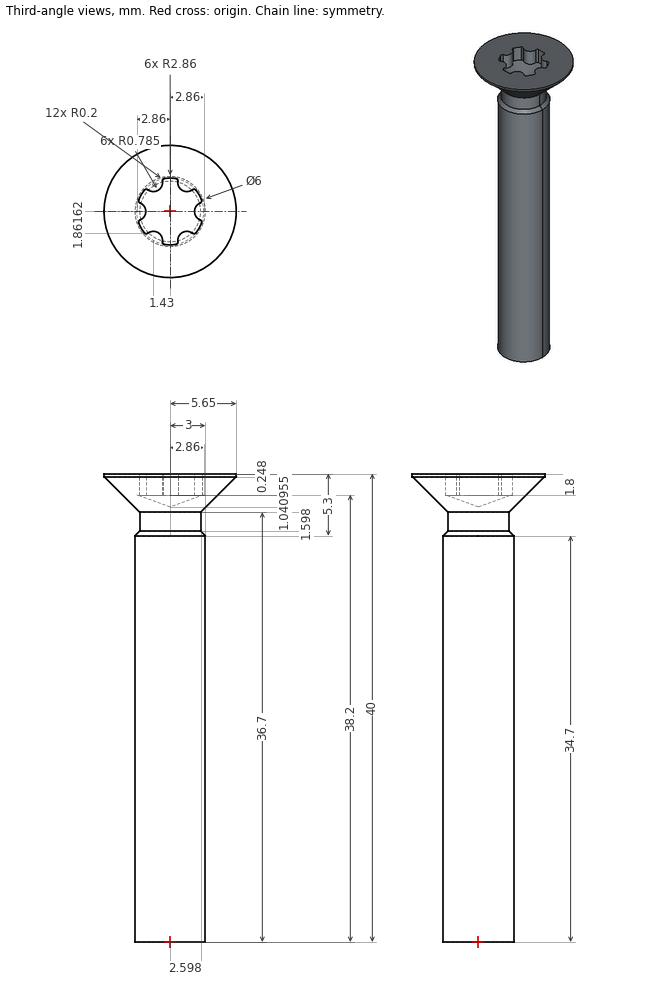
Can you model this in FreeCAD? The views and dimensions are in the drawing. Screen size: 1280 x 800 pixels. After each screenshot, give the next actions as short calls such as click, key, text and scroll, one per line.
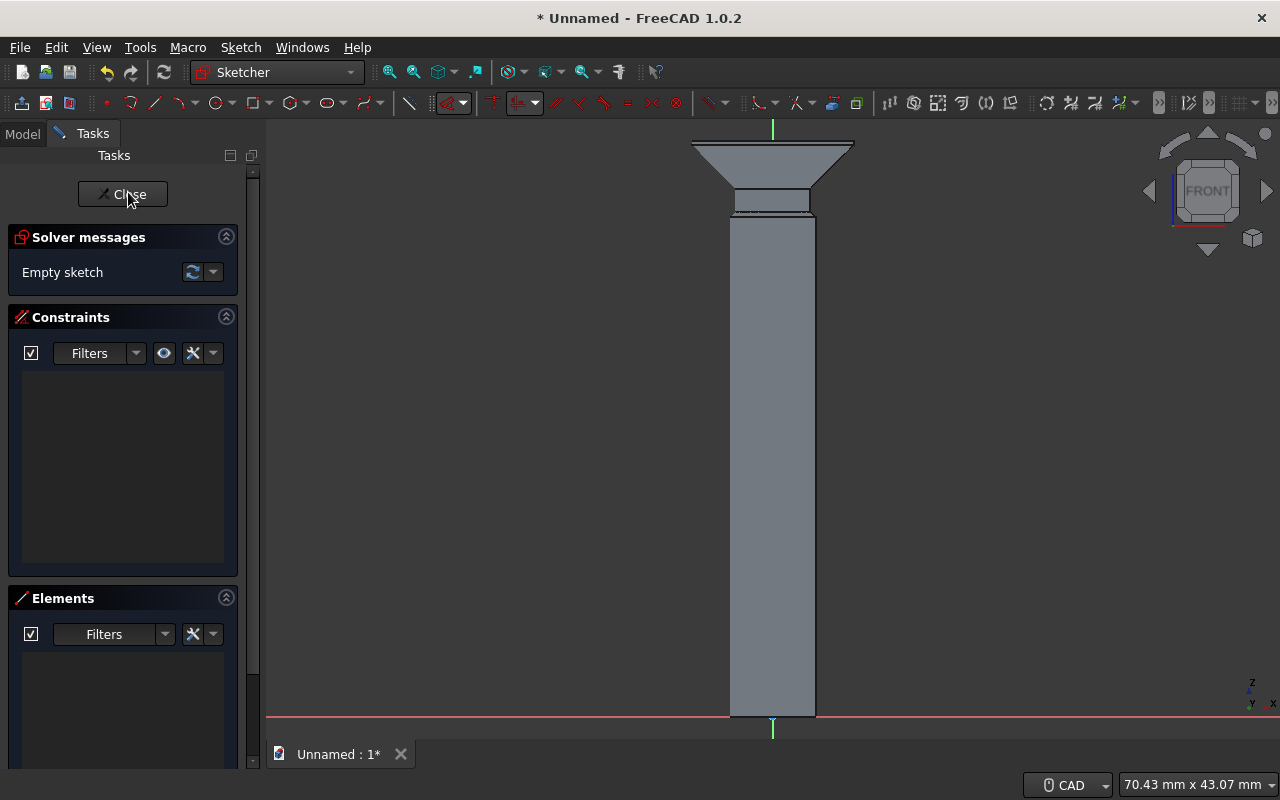
click(70, 104)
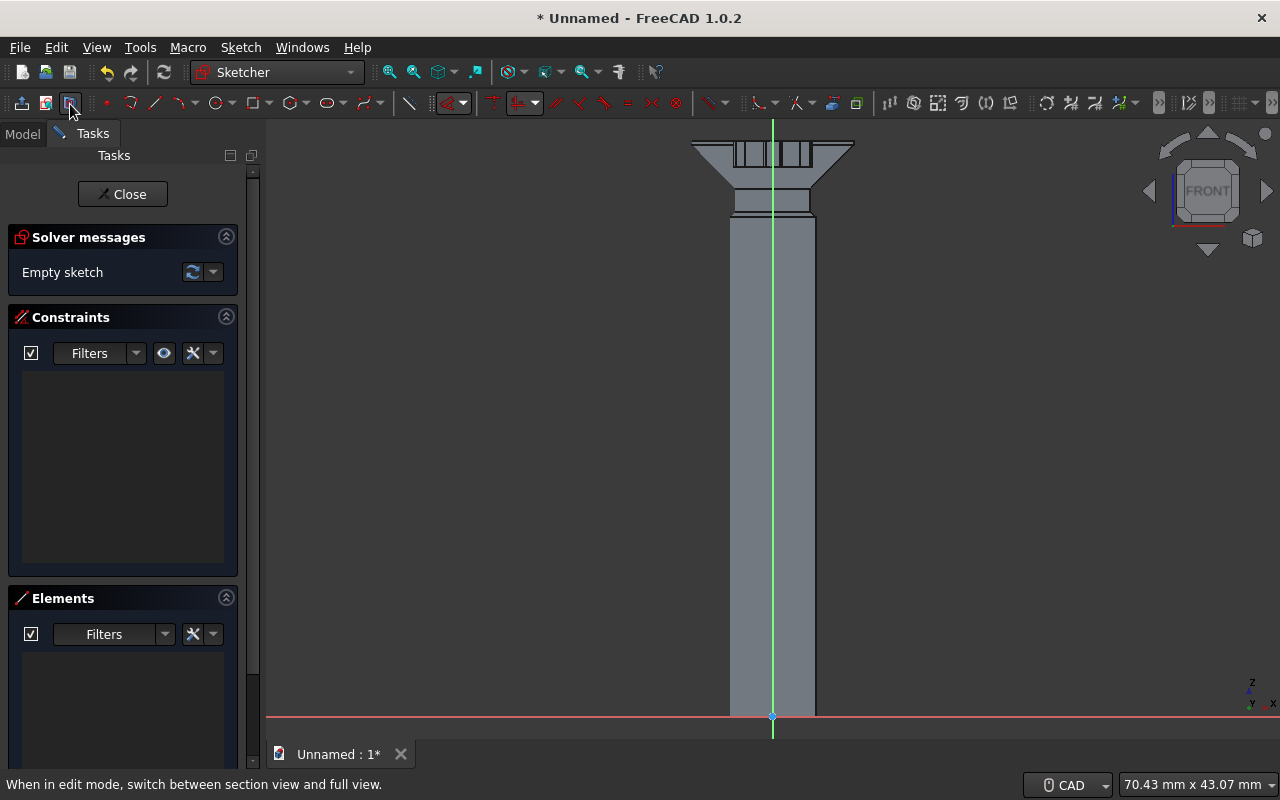
scroll(801, 154, up, 13)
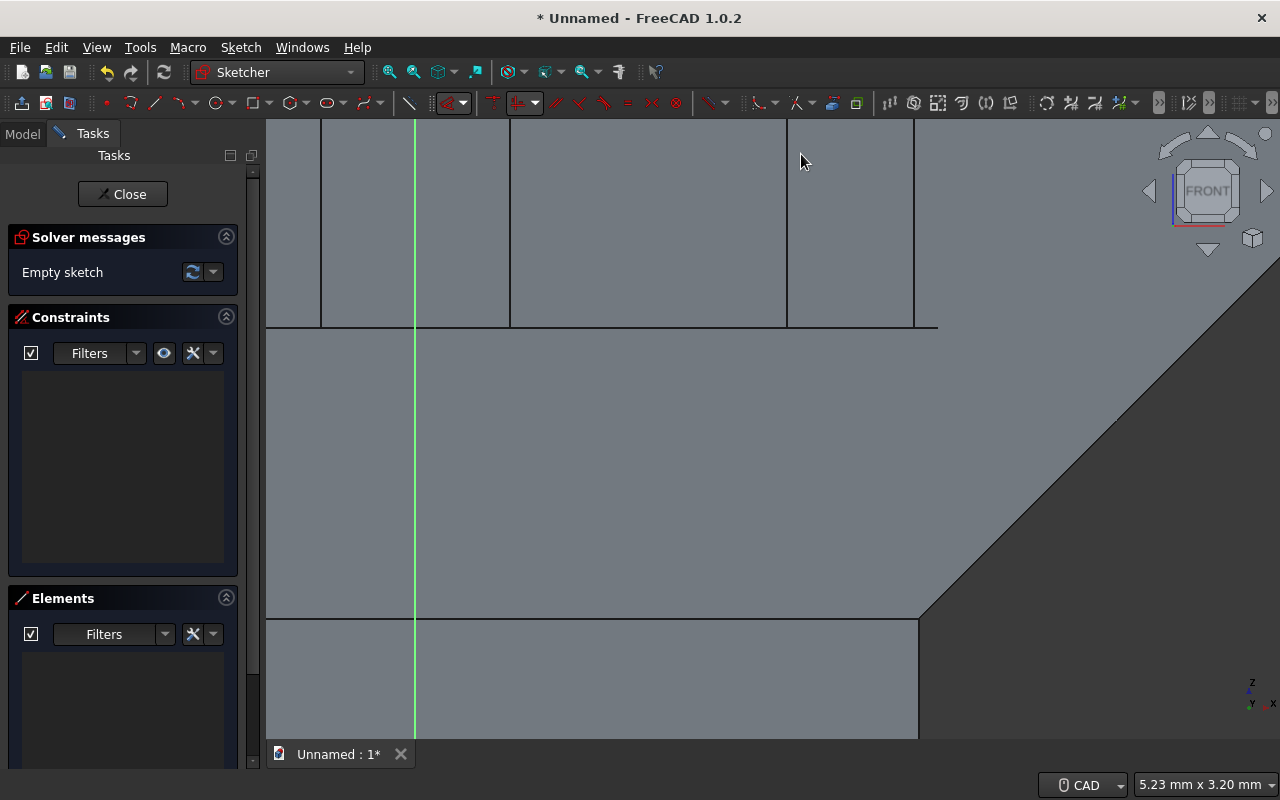
key(g)
key(m)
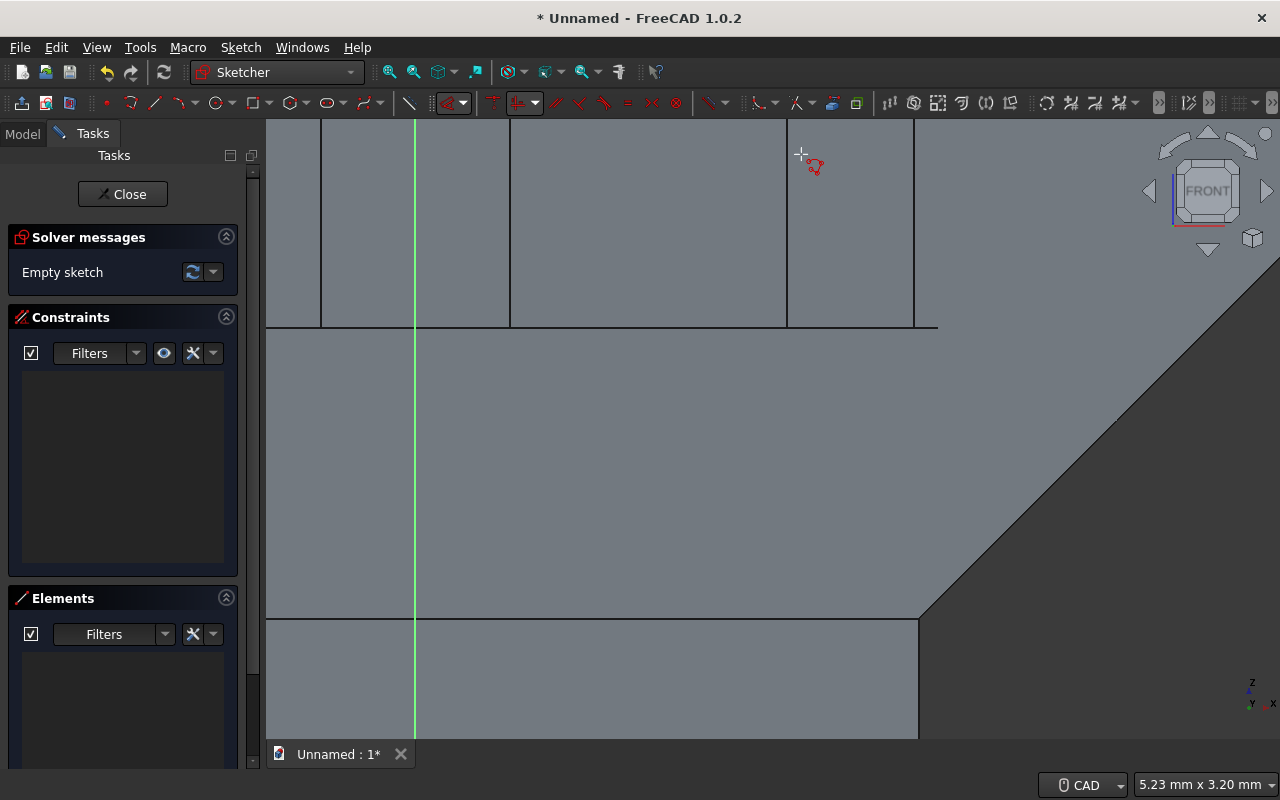
click(415, 530)
click(424, 328)
click(970, 328)
click(415, 531)
key(Escape)
key(Escape)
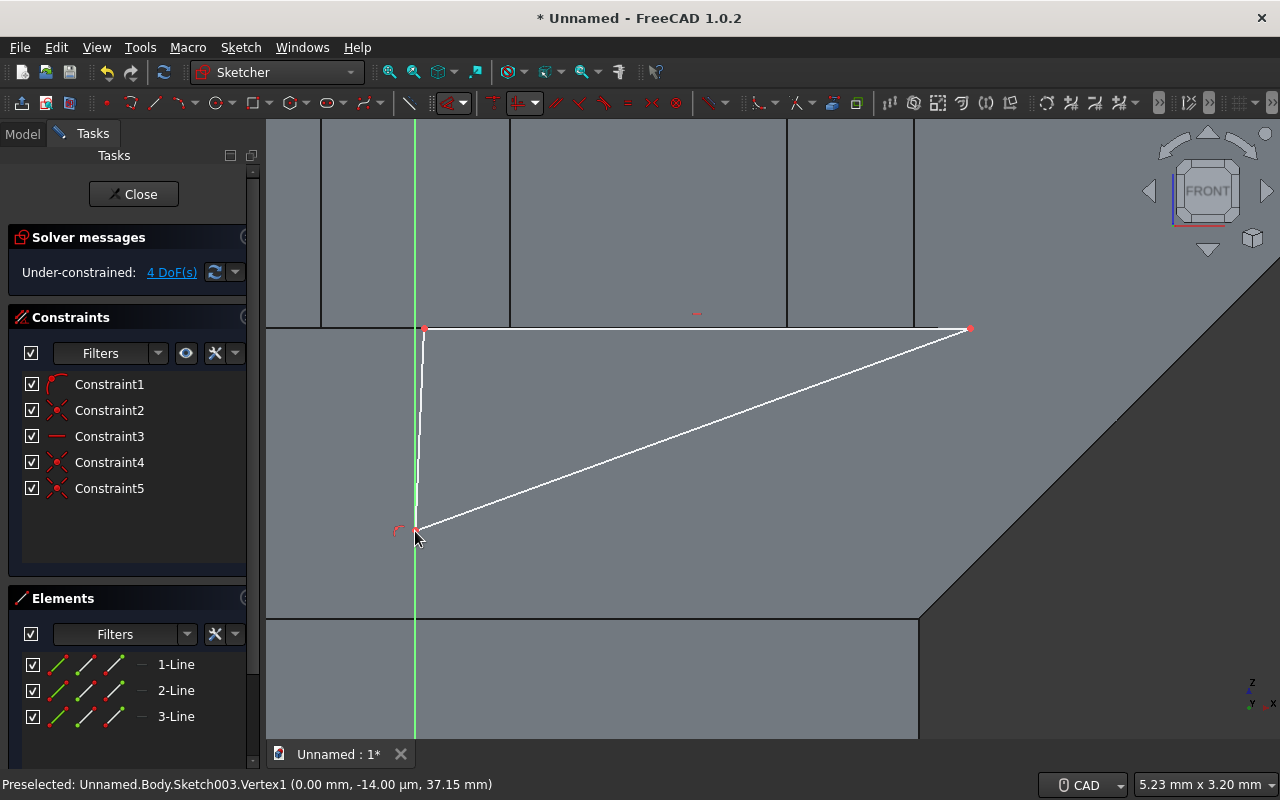
click(418, 470)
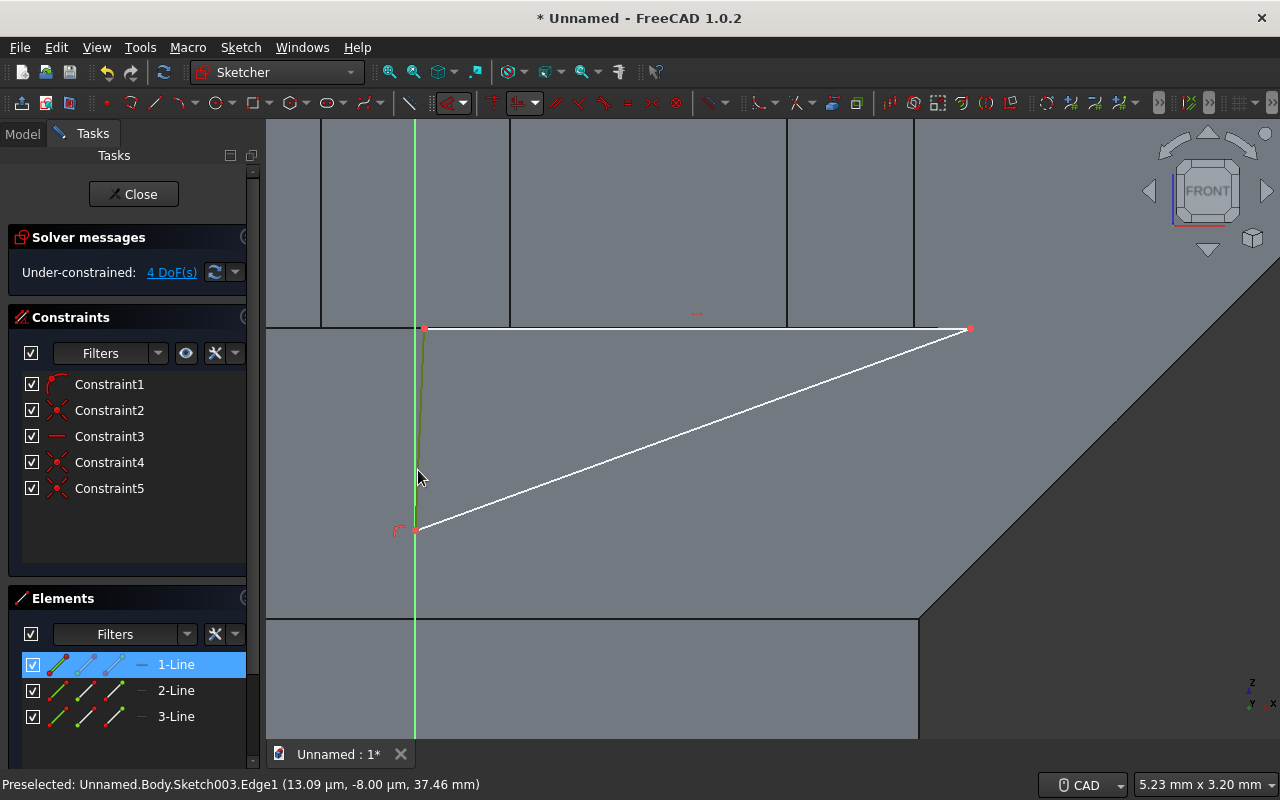
click(538, 104)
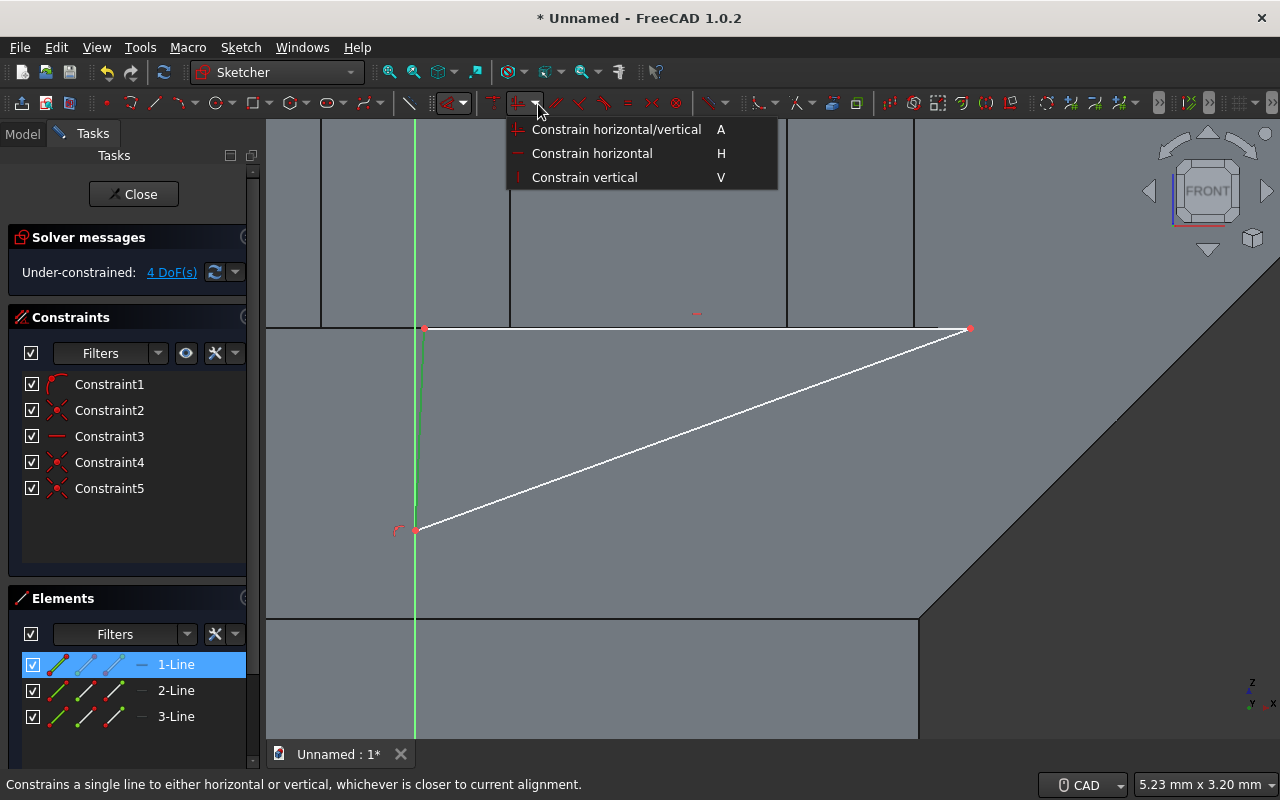
click(642, 177)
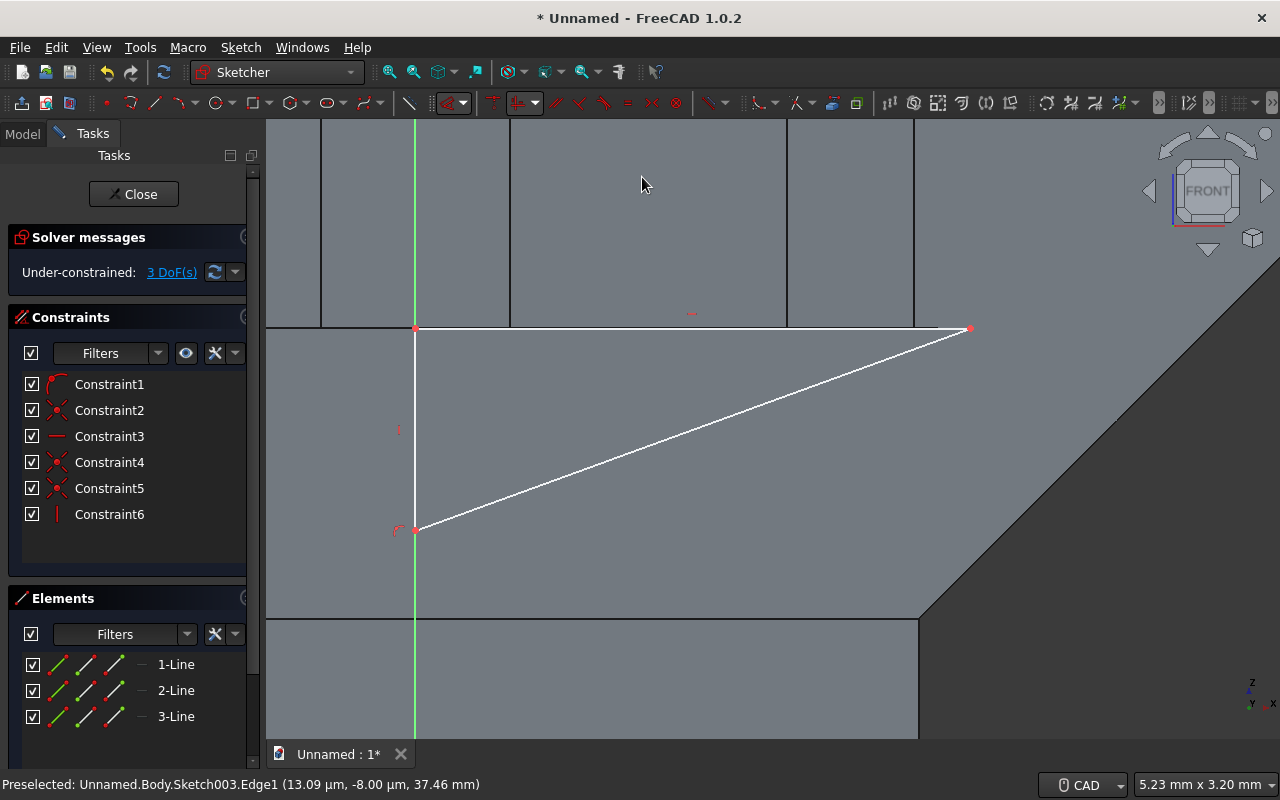
click(582, 329)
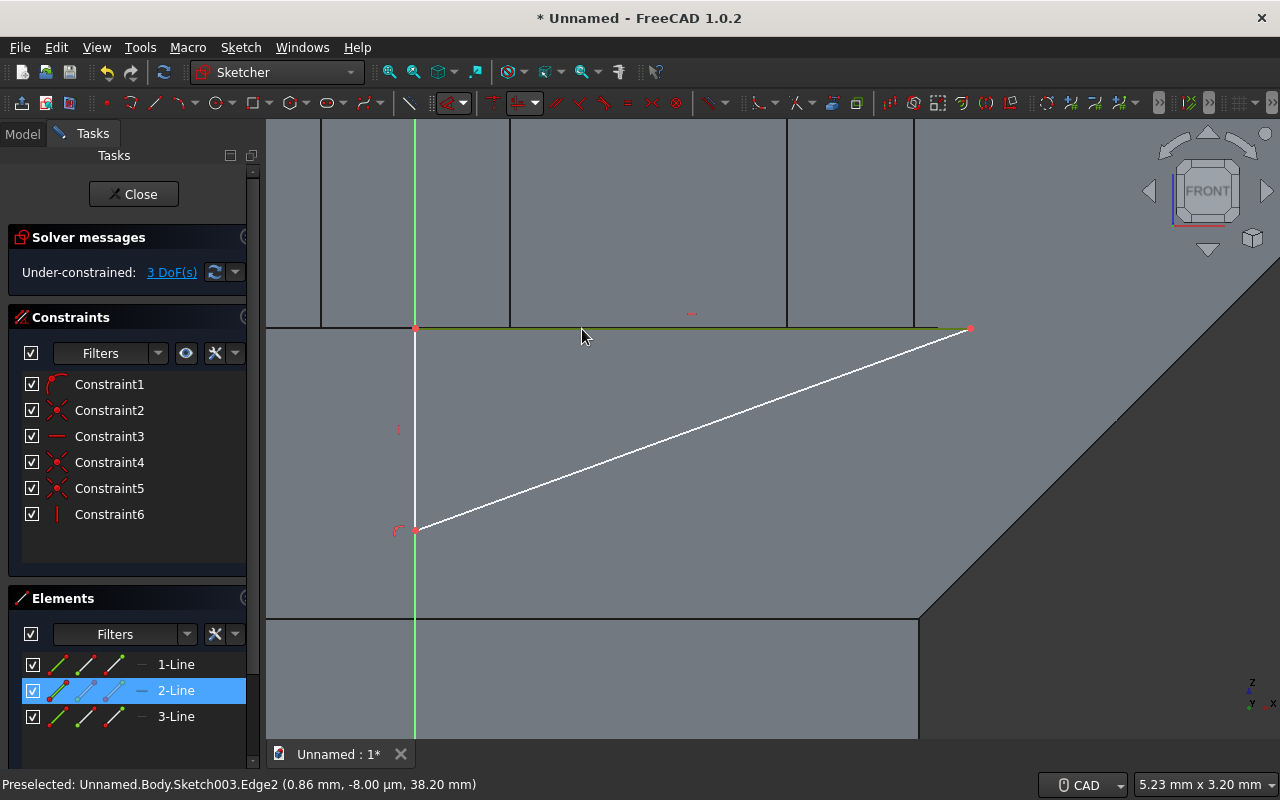
key(l)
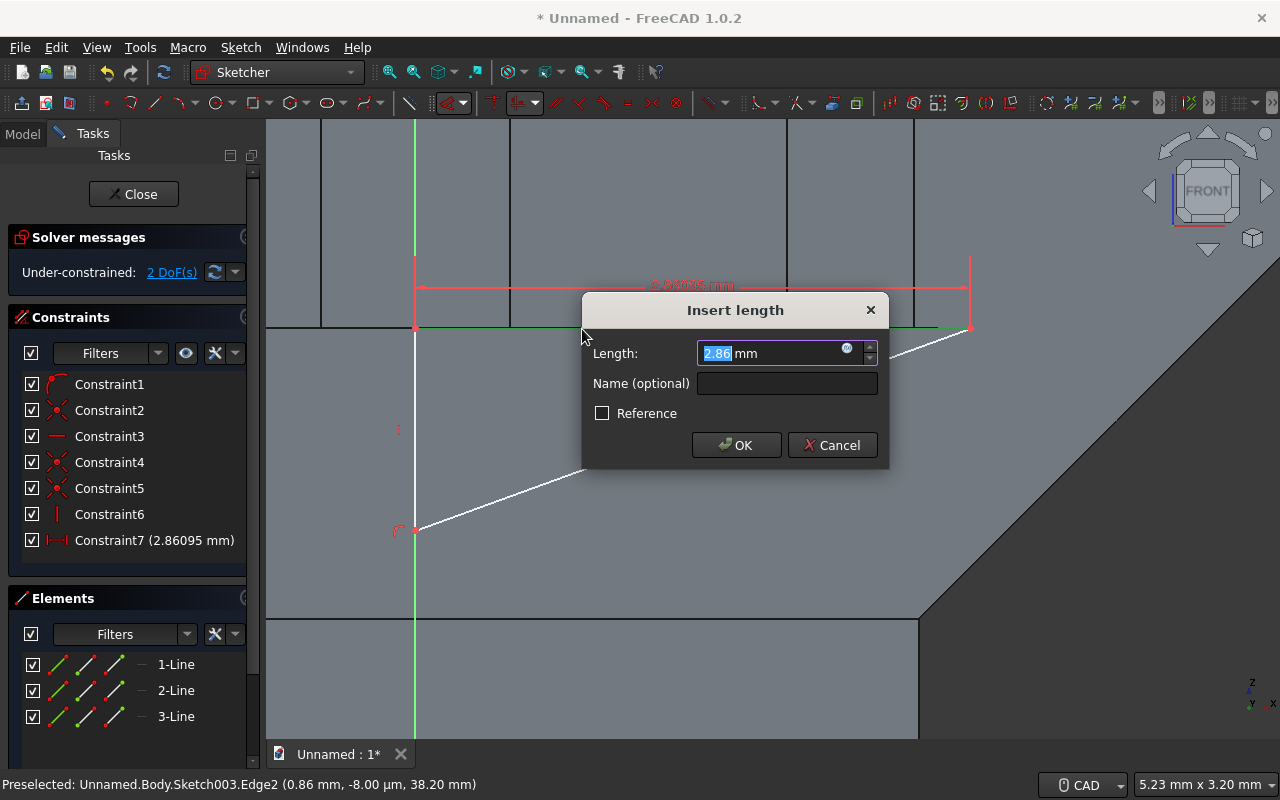
text(2.86)
key(Return)